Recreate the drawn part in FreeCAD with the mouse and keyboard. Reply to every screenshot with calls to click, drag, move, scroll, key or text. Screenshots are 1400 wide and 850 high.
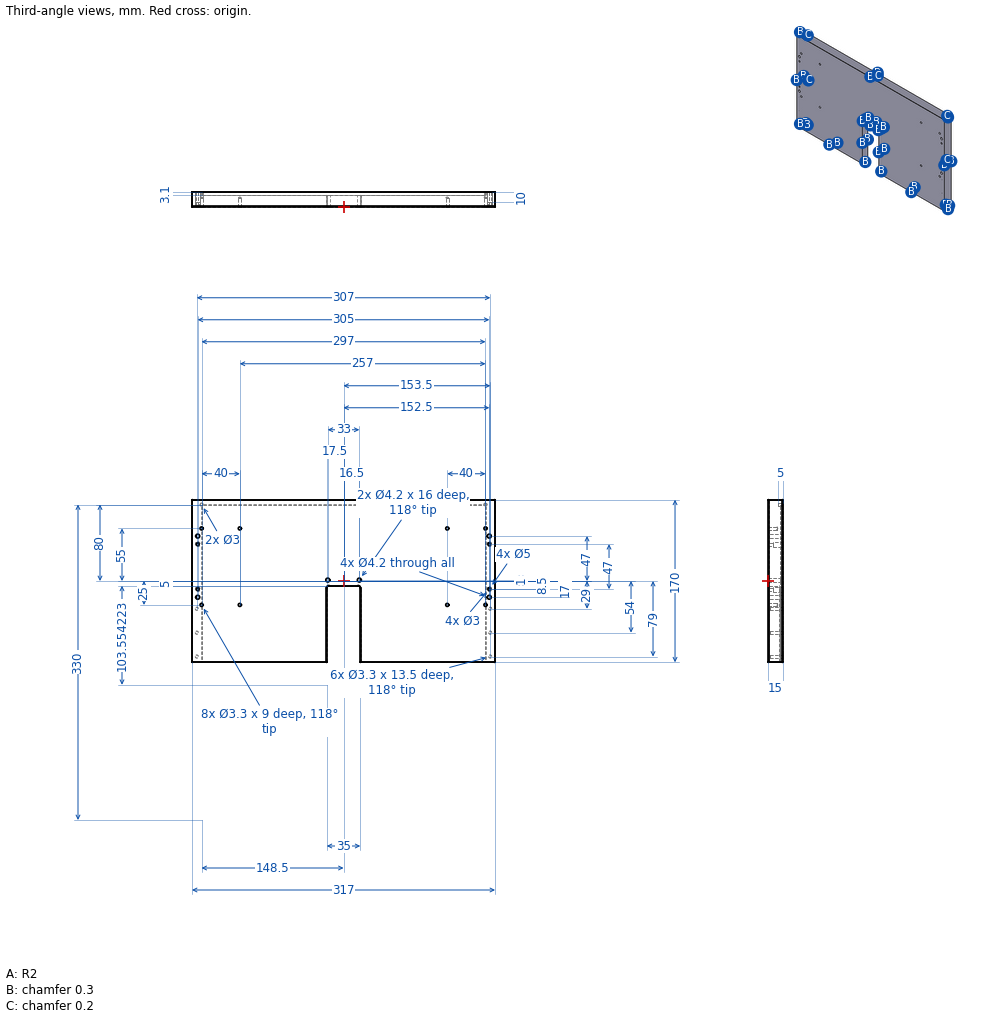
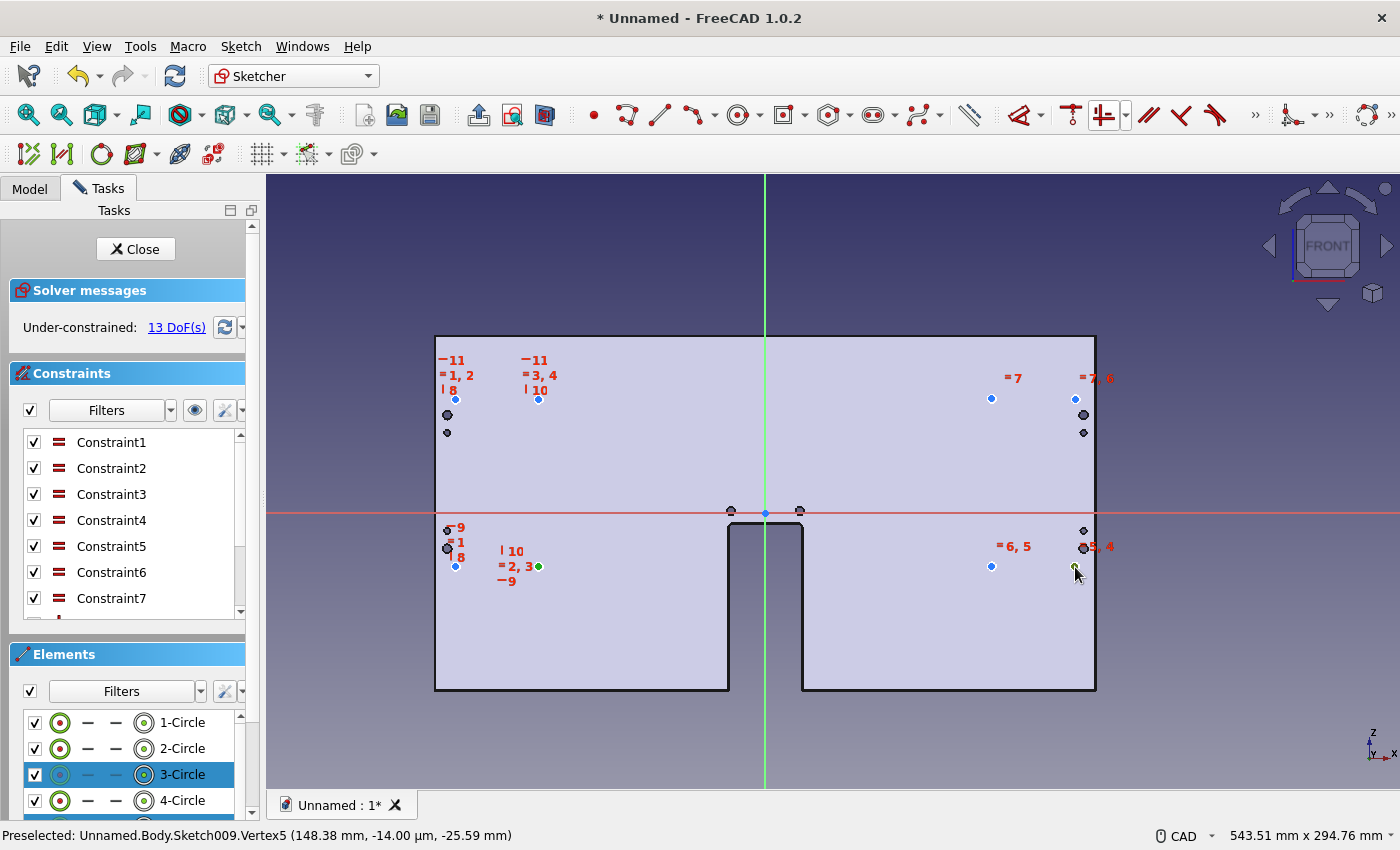
key(h)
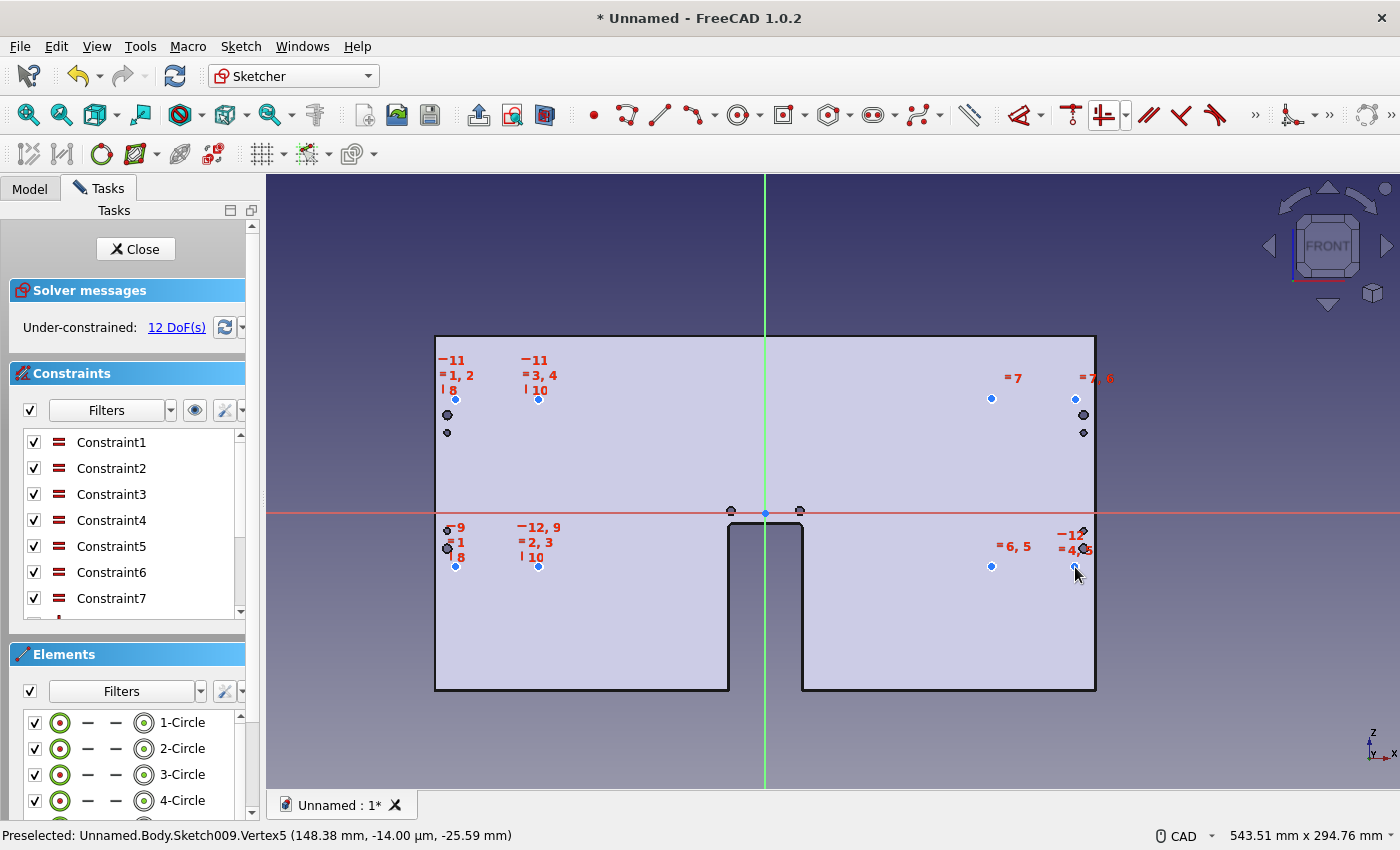
click(1075, 567)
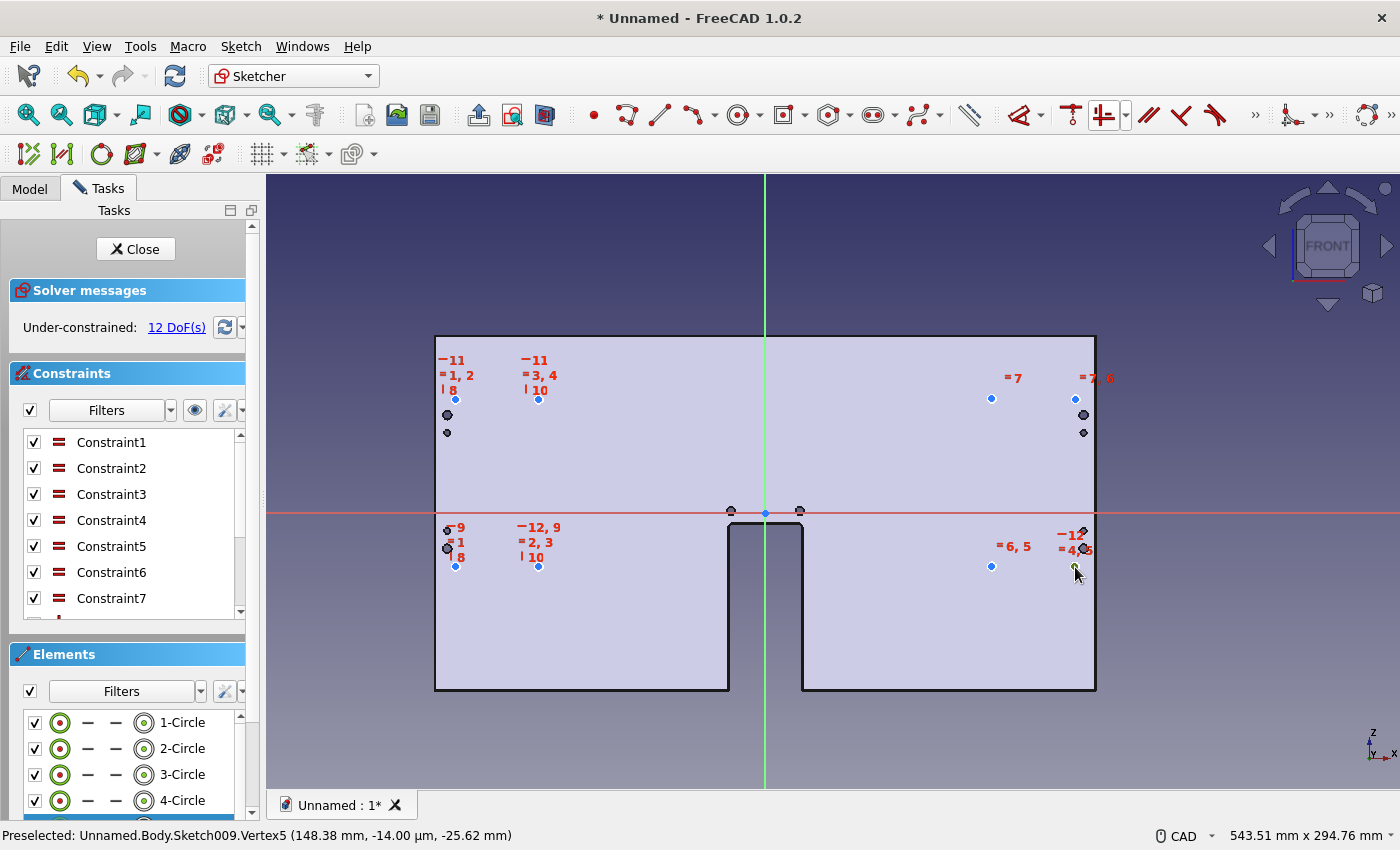
click(992, 566)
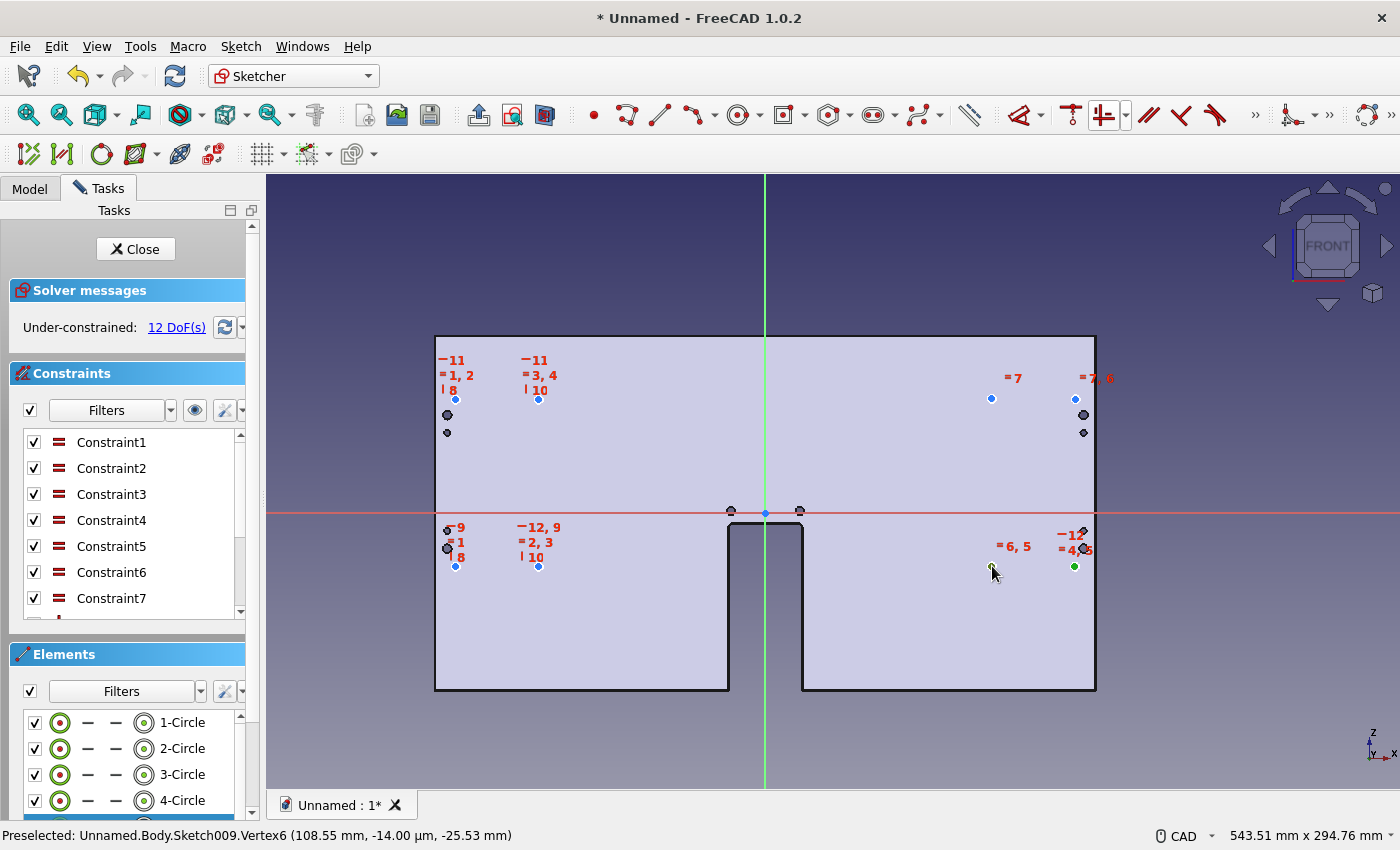
key(h)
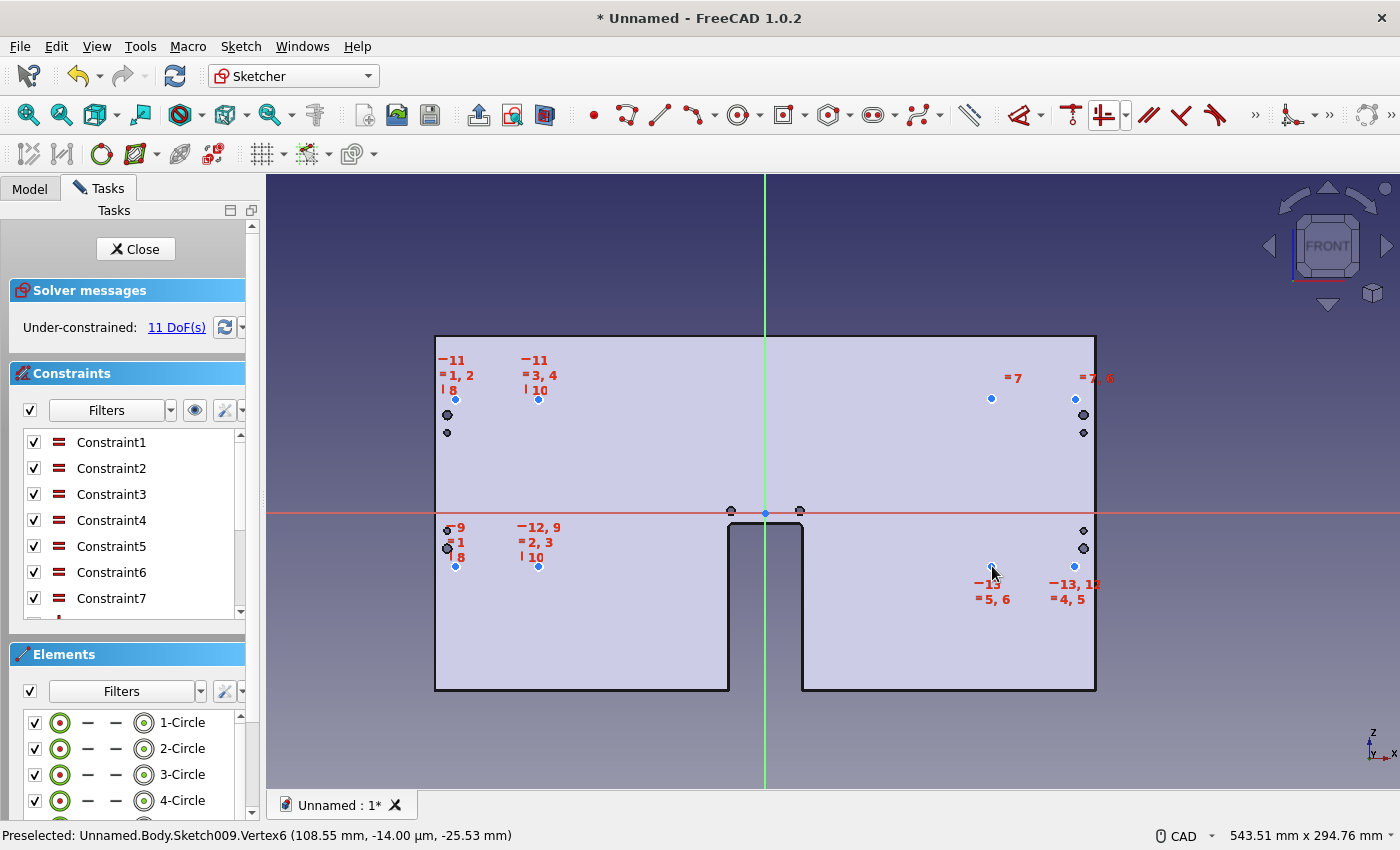
click(1075, 567)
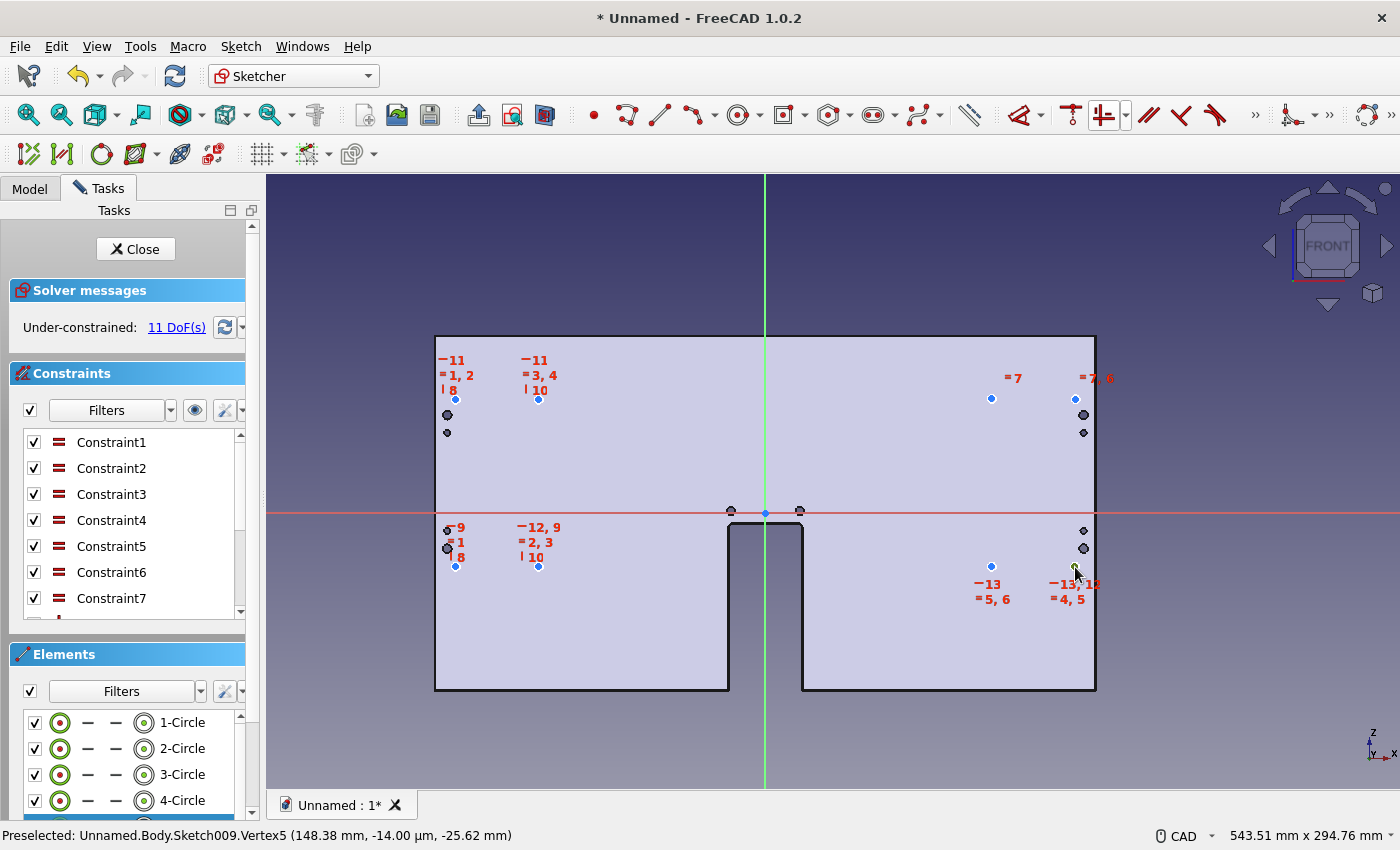
click(1076, 399)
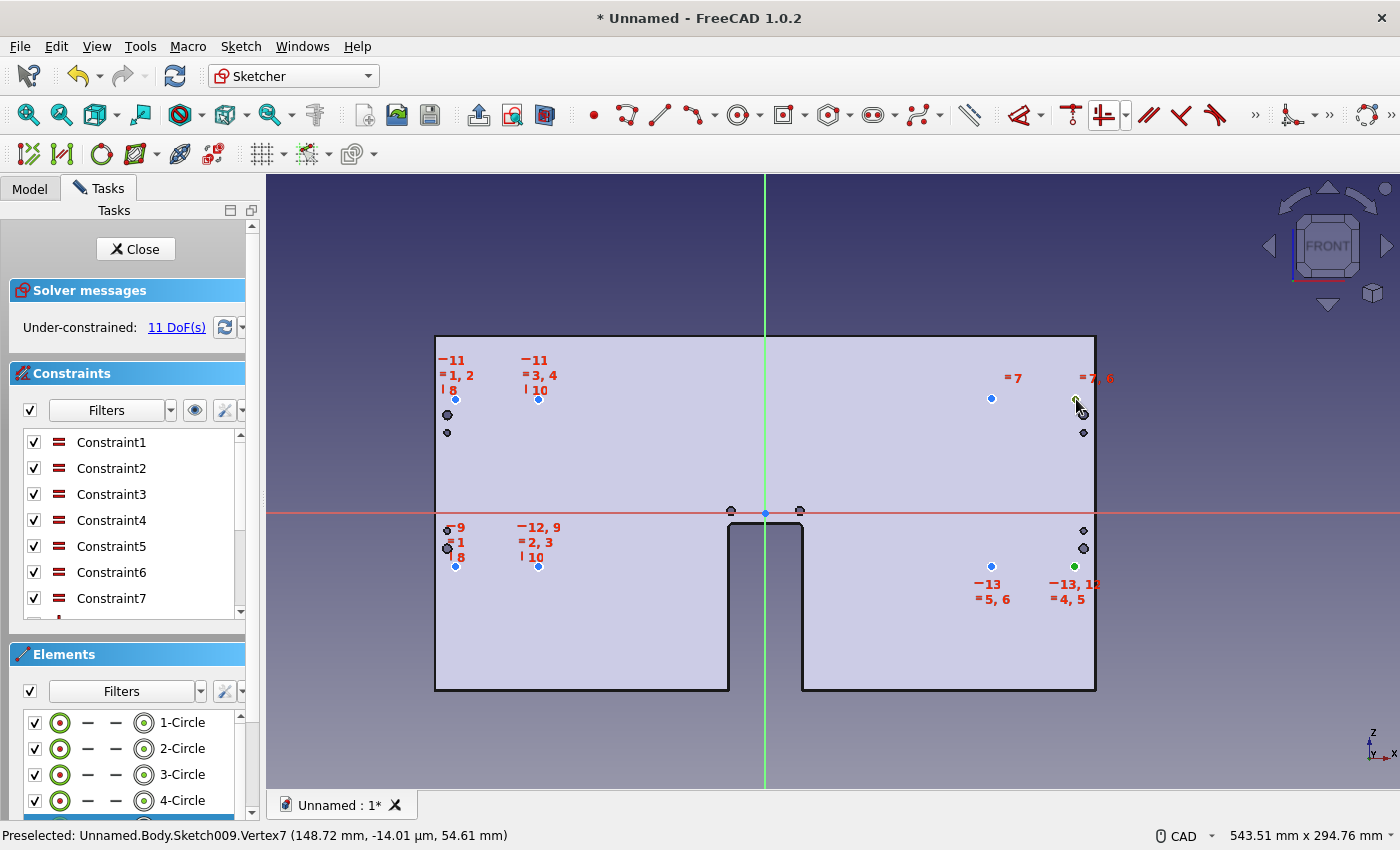
click(1126, 116)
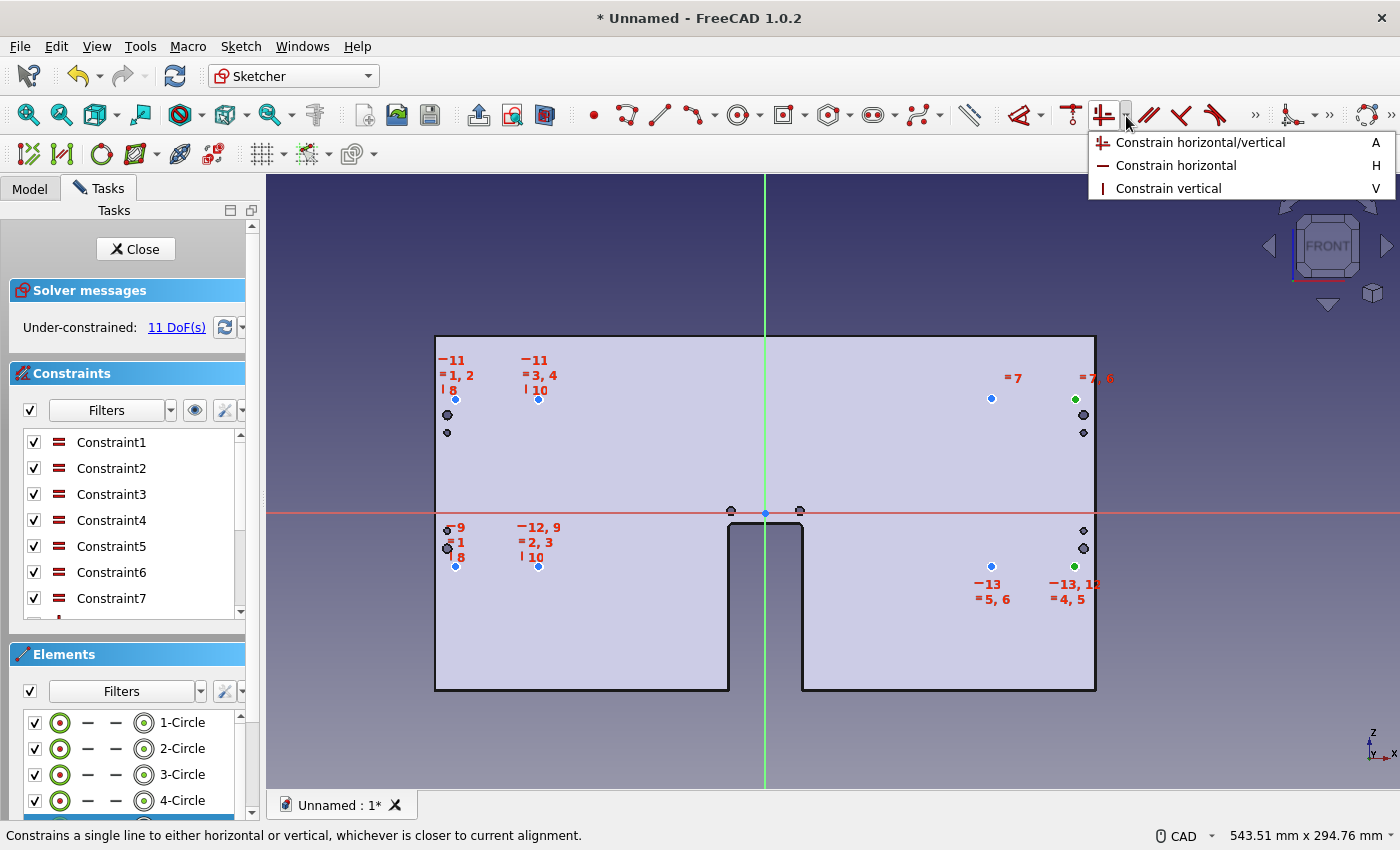
click(1242, 188)